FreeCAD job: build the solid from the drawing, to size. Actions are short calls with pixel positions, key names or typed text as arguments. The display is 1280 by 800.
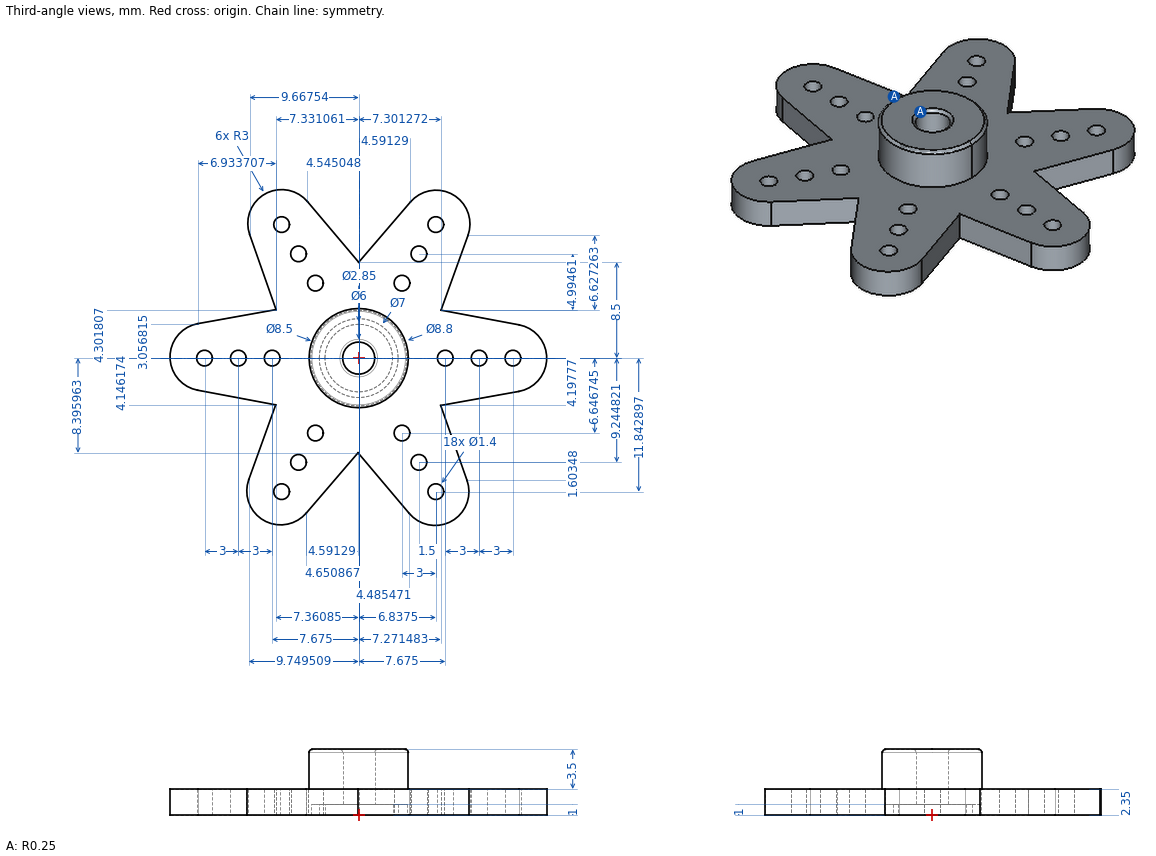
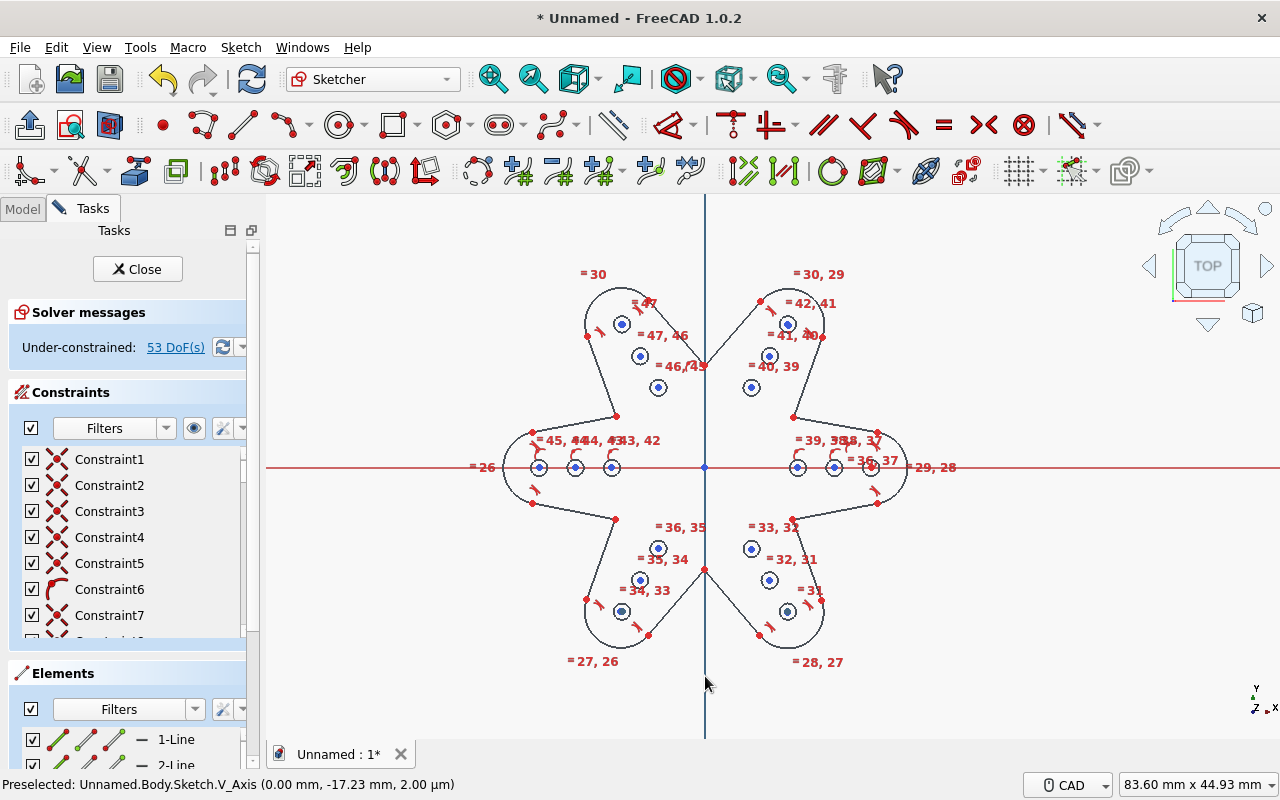
click(984, 126)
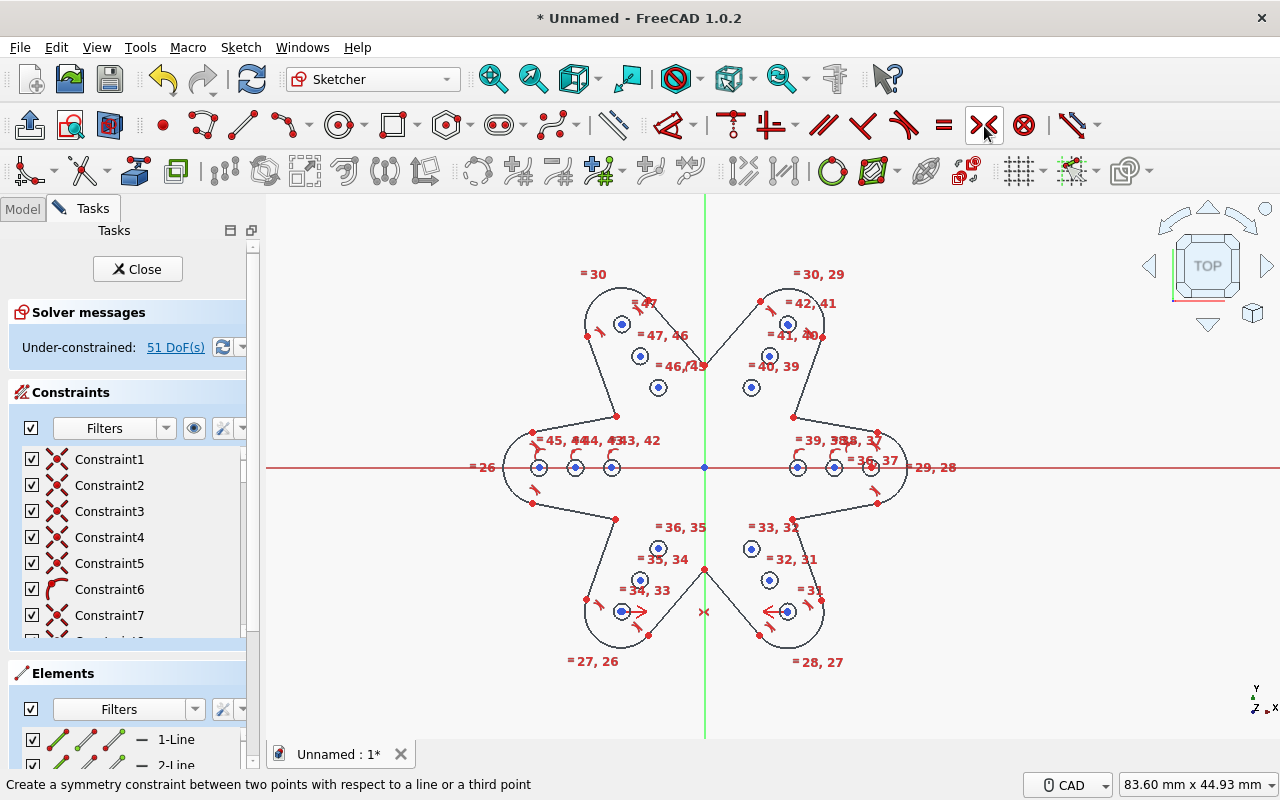
click(770, 580)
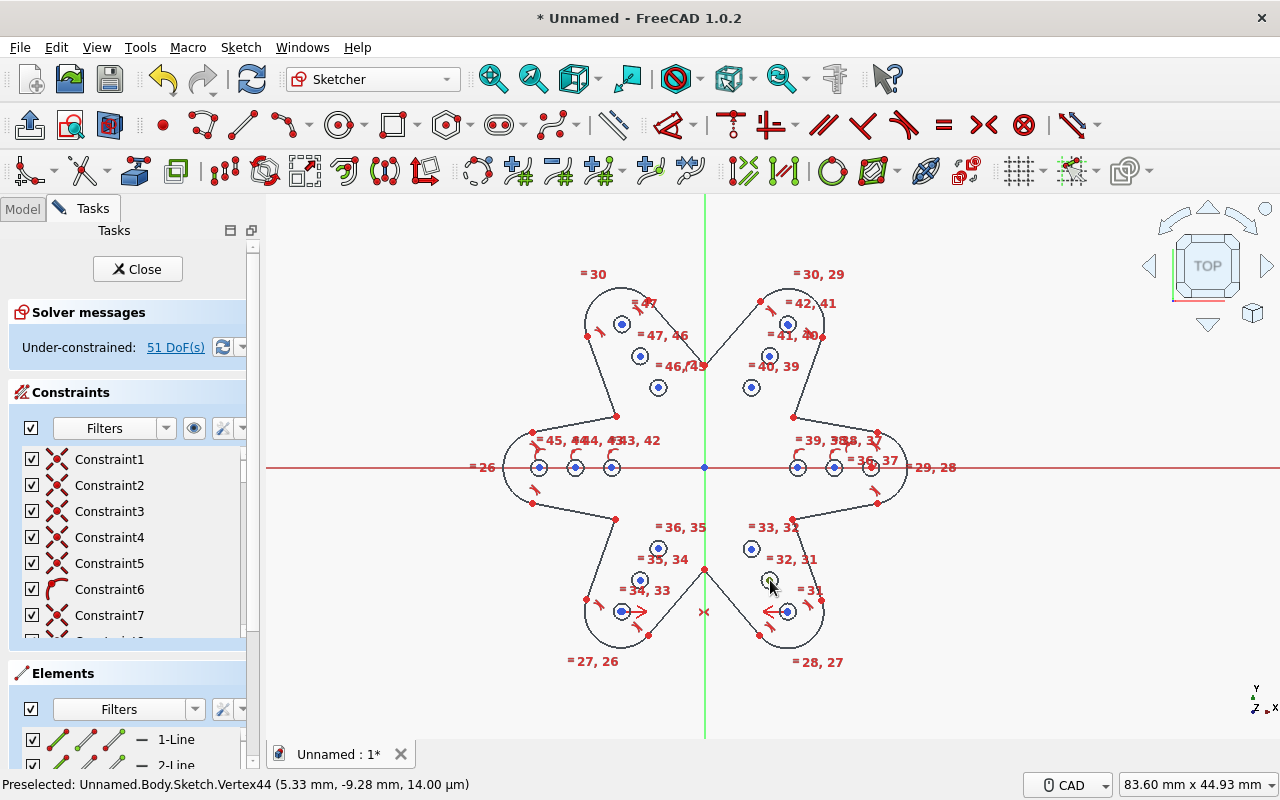
click(640, 580)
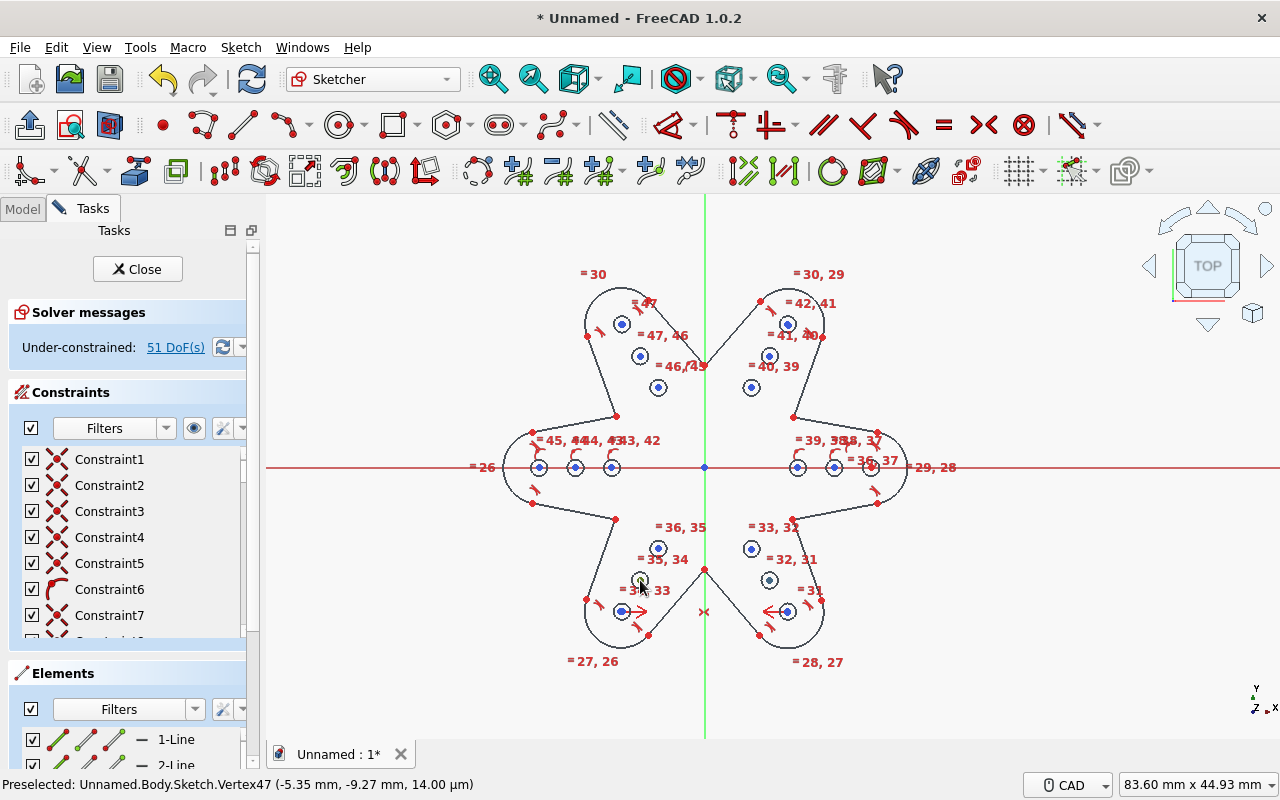
click(705, 676)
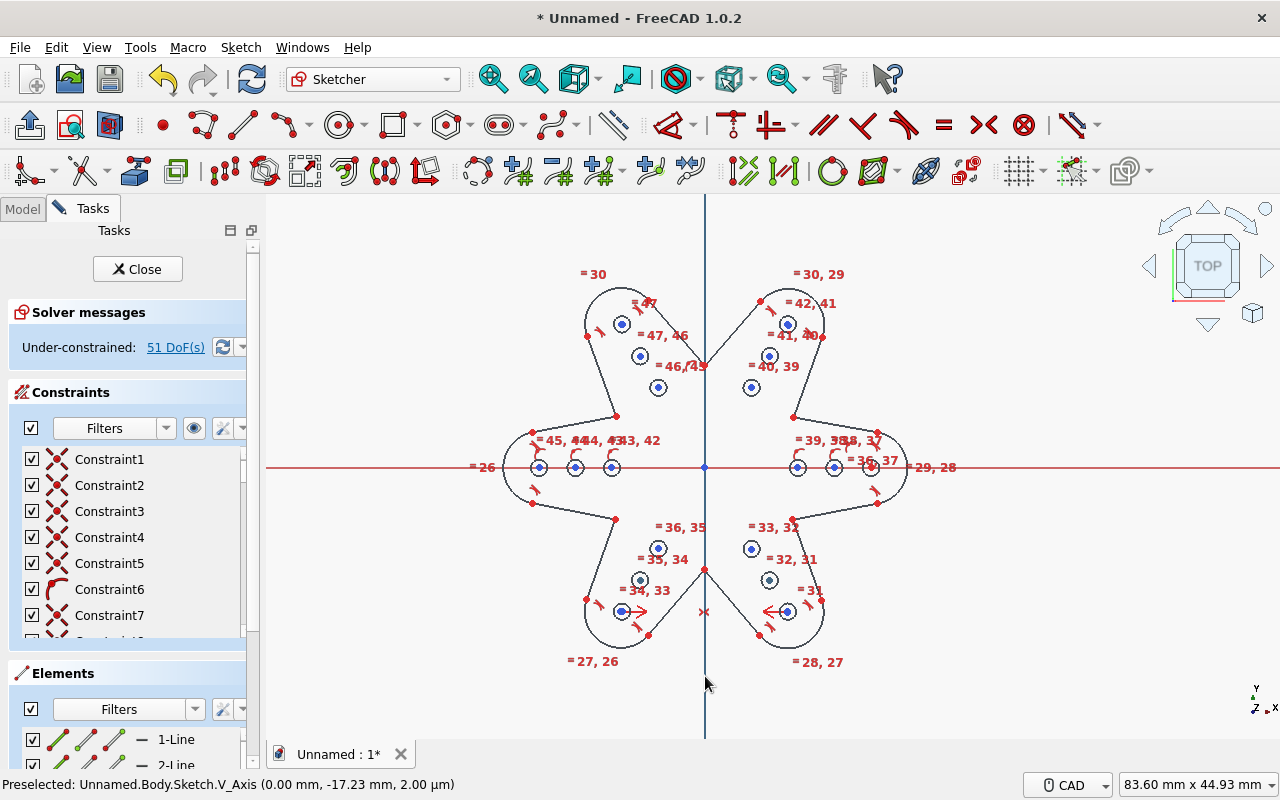
click(984, 126)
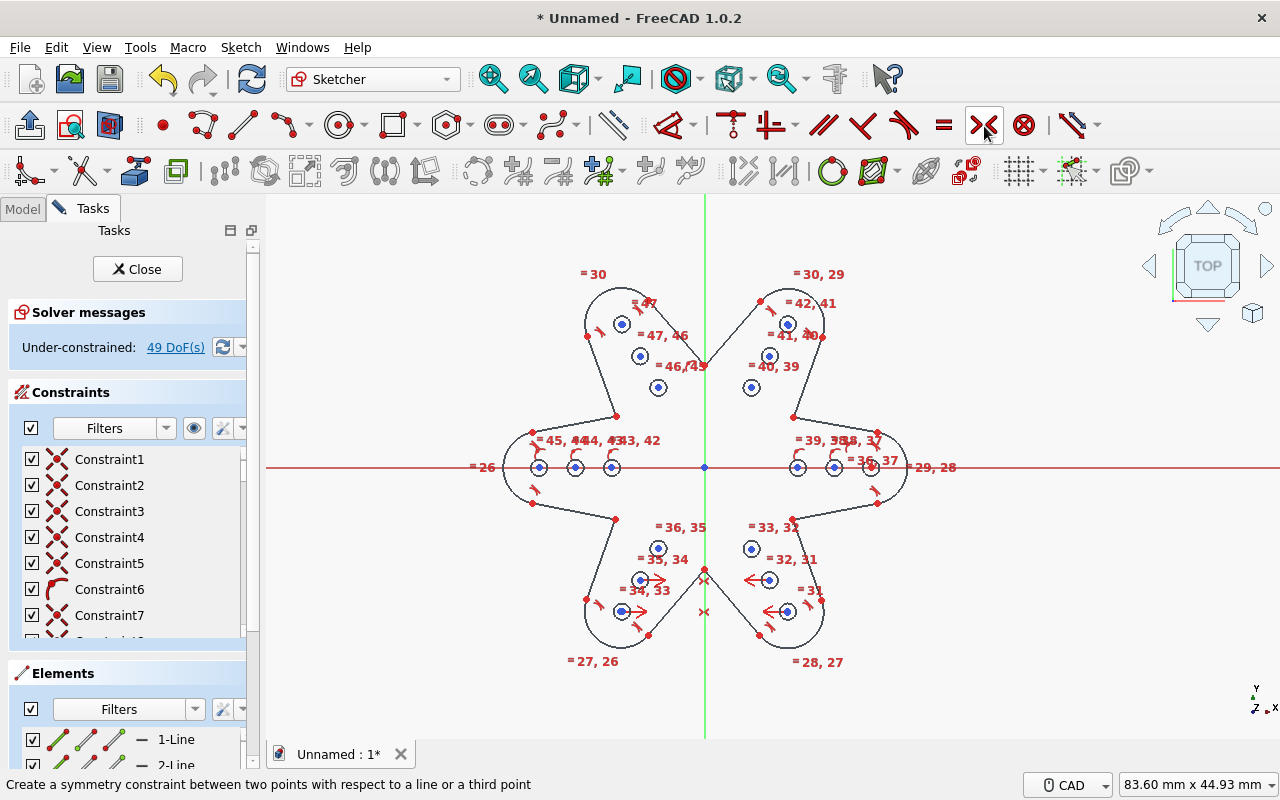
click(752, 549)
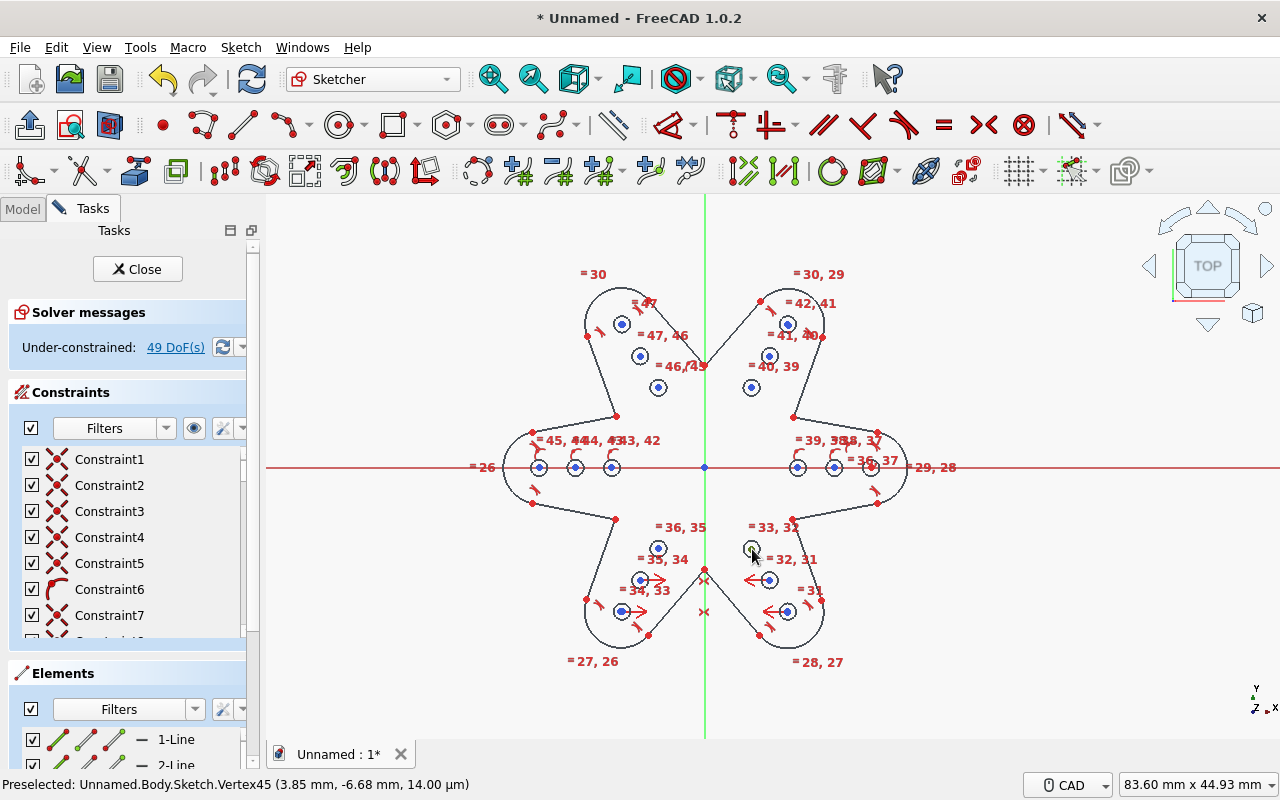
click(658, 549)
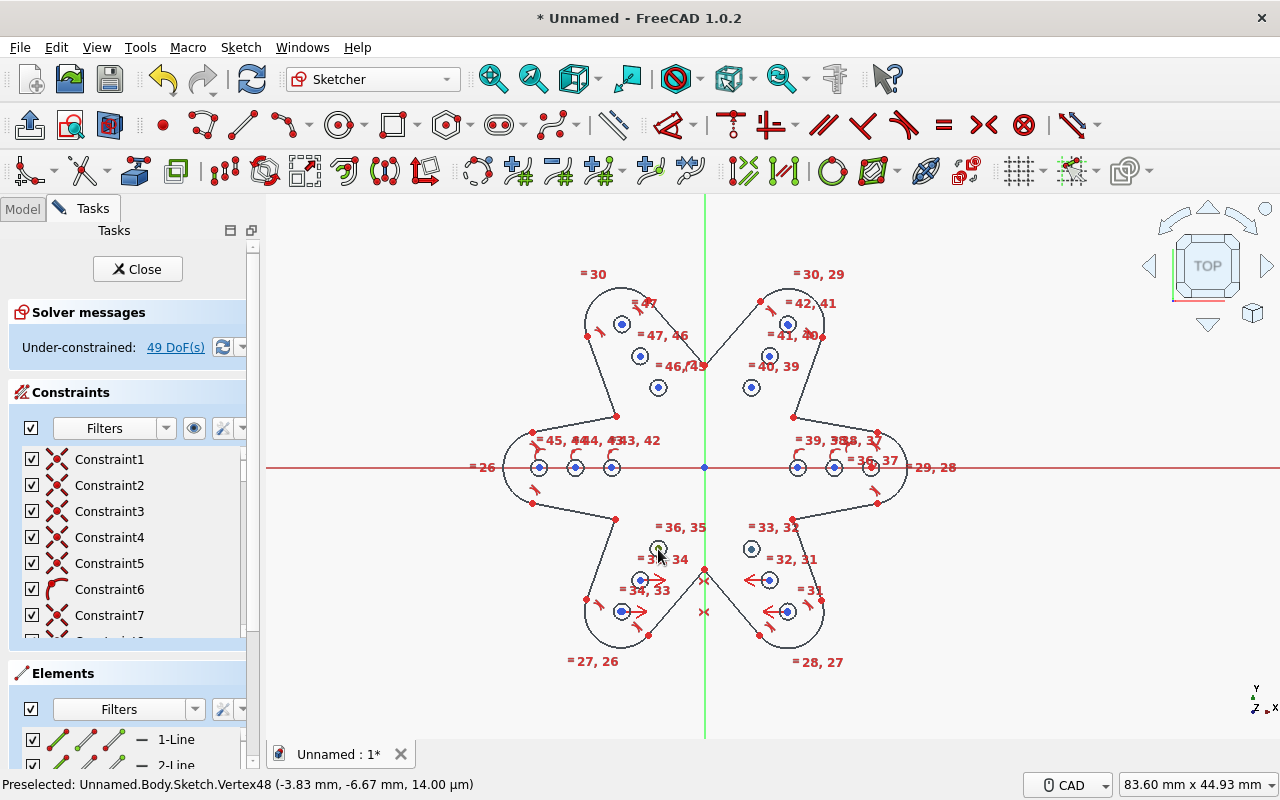
click(705, 676)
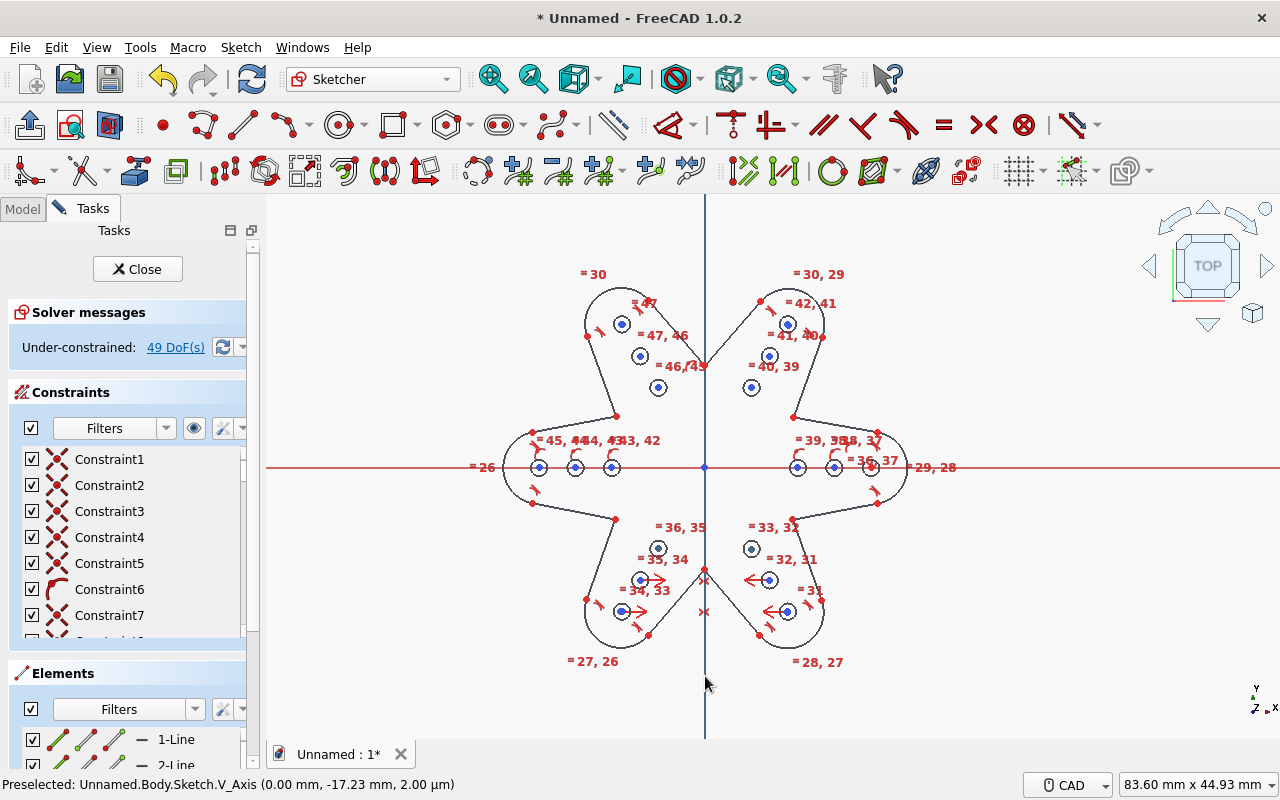
click(984, 126)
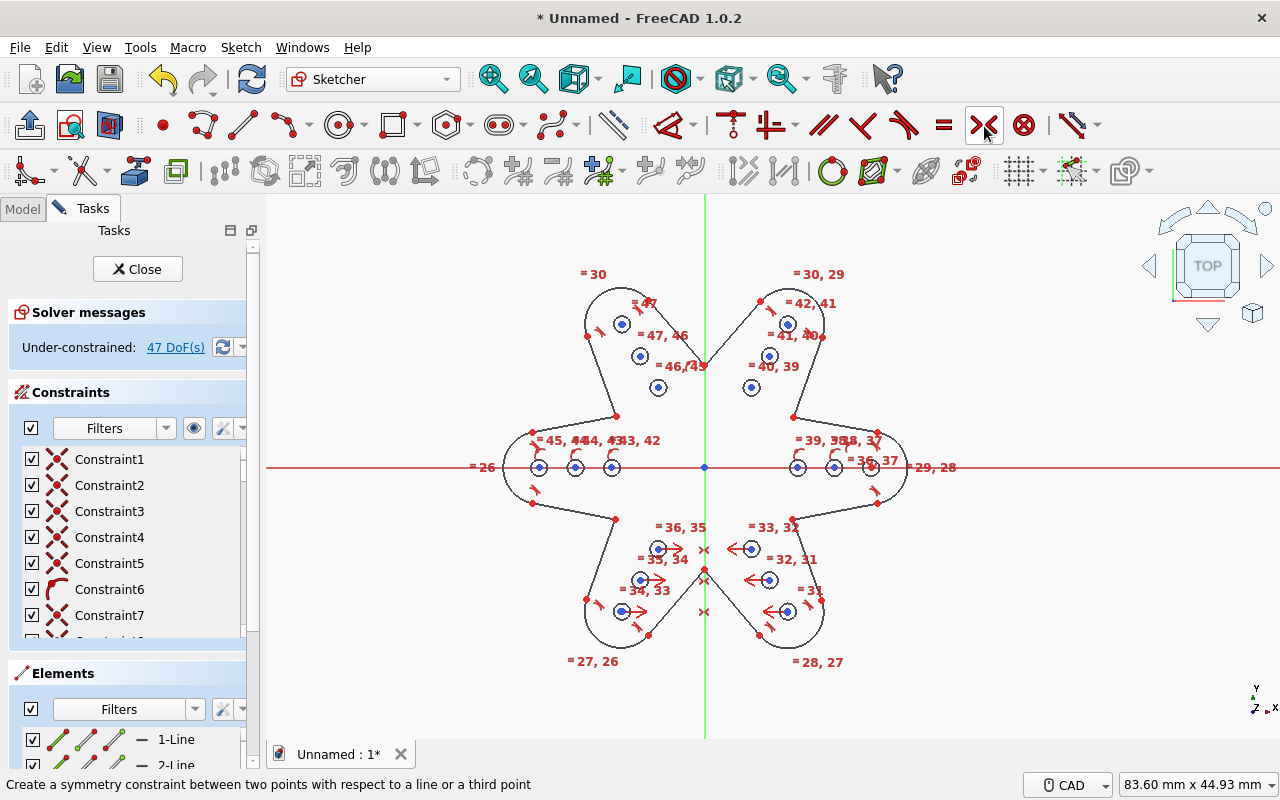
click(752, 549)